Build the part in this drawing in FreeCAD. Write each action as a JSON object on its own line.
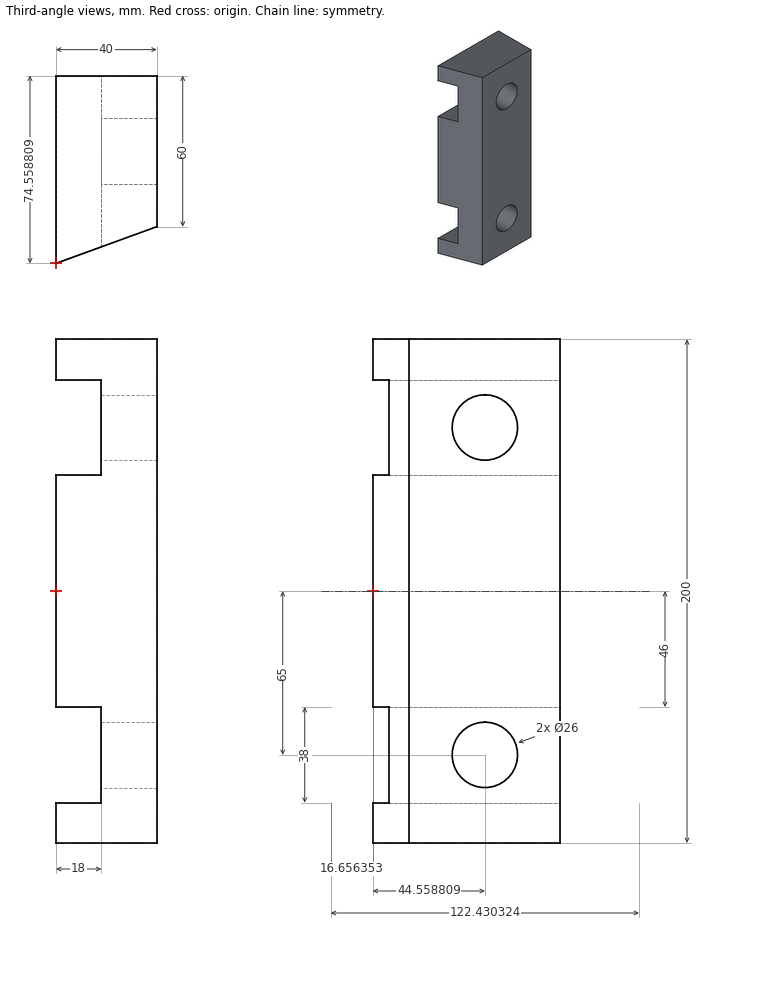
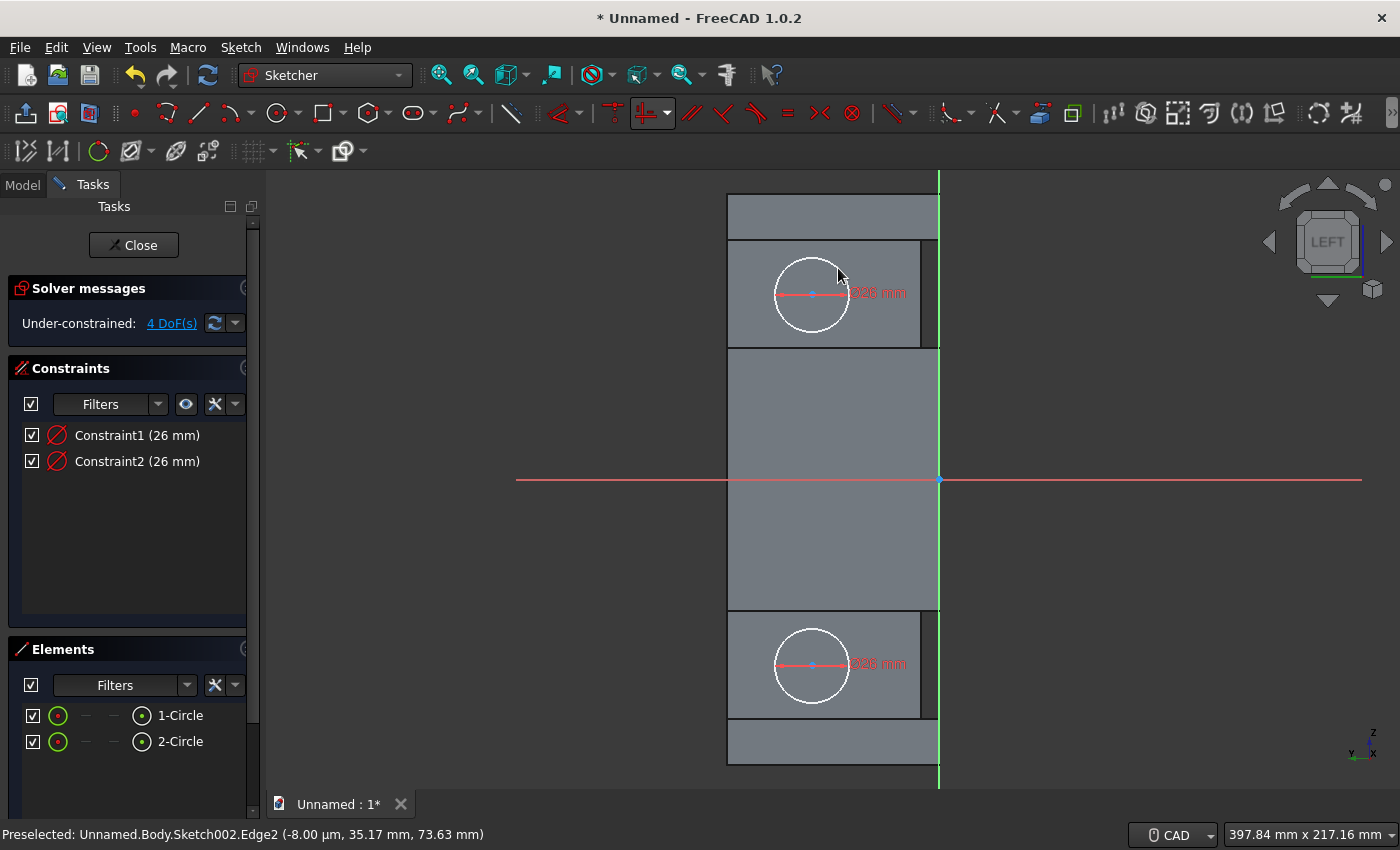
{"action": "left_click", "coordinate": [812, 666]}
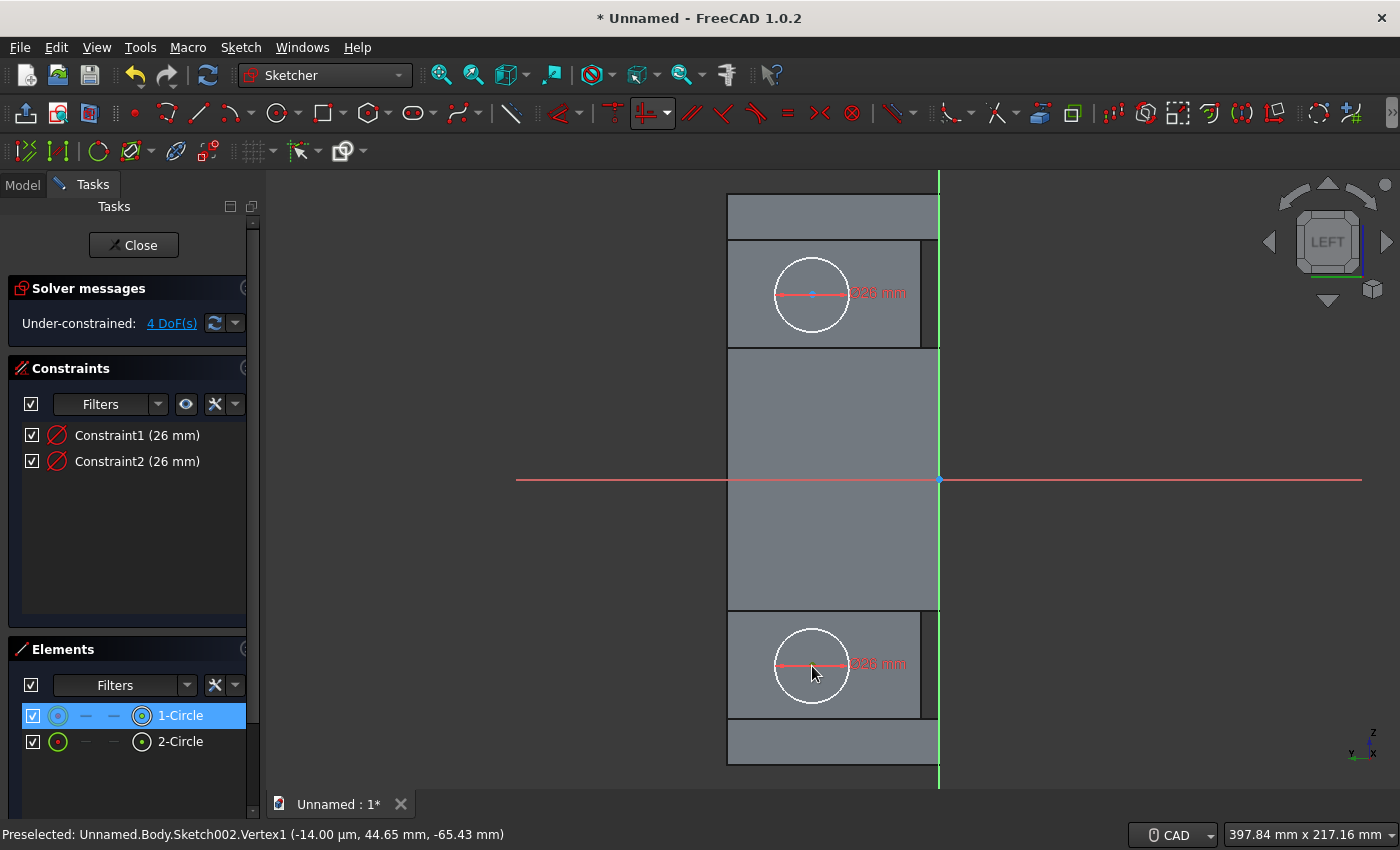
{"action": "left_click", "coordinate": [812, 295]}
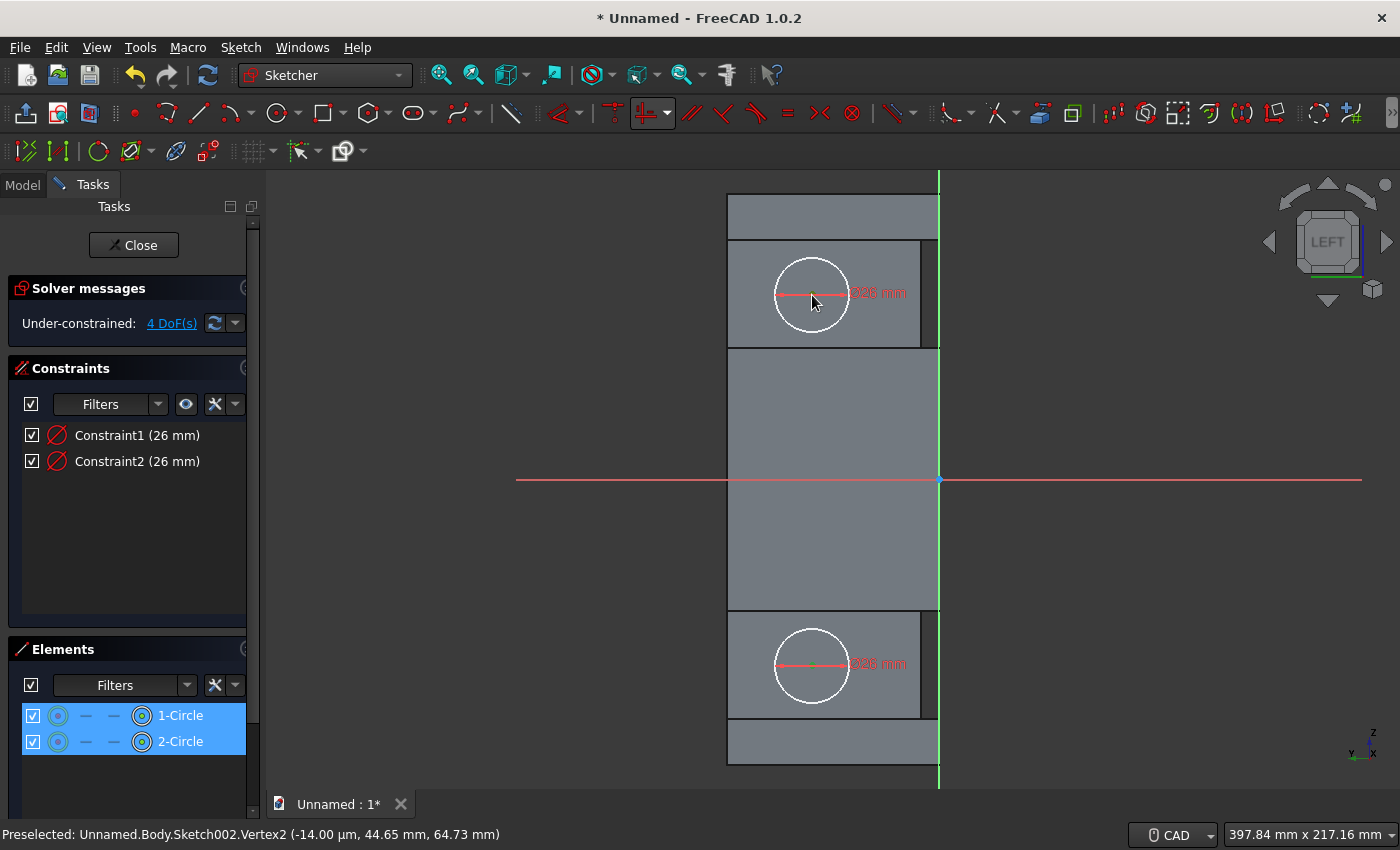
{"action": "left_click", "coordinate": [563, 480]}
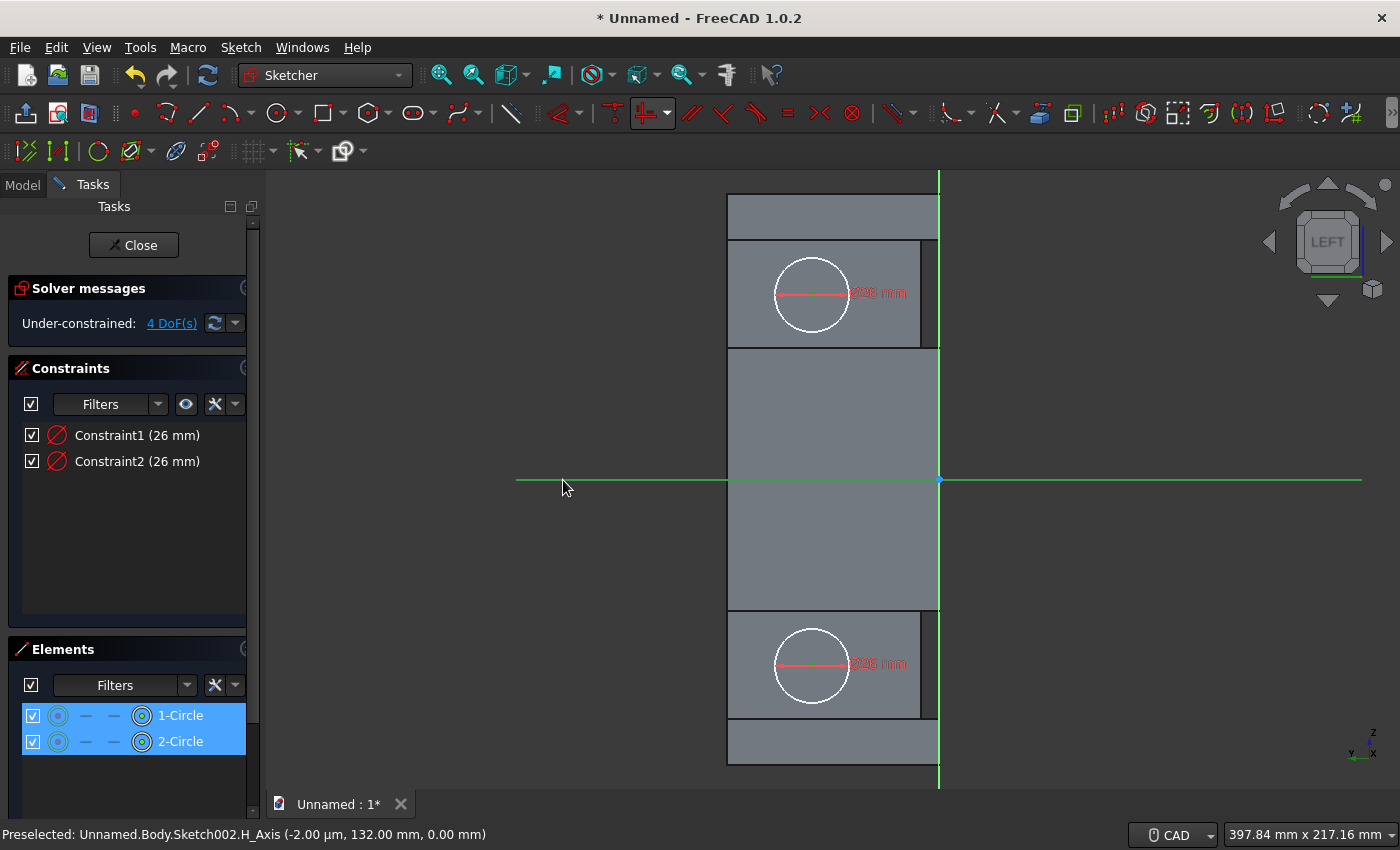
{"action": "left_click", "coordinate": [820, 114]}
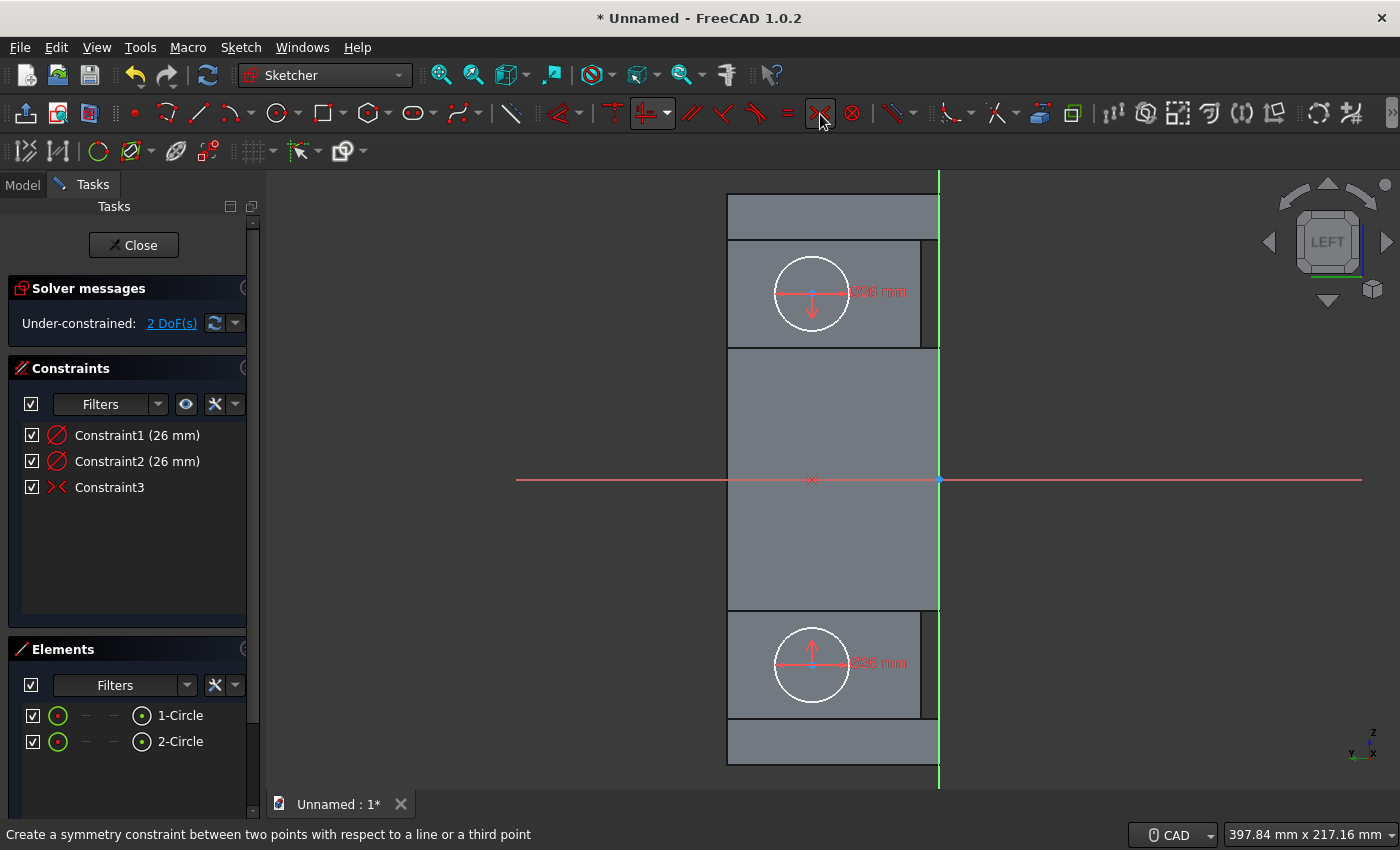
{"action": "left_click", "coordinate": [558, 114]}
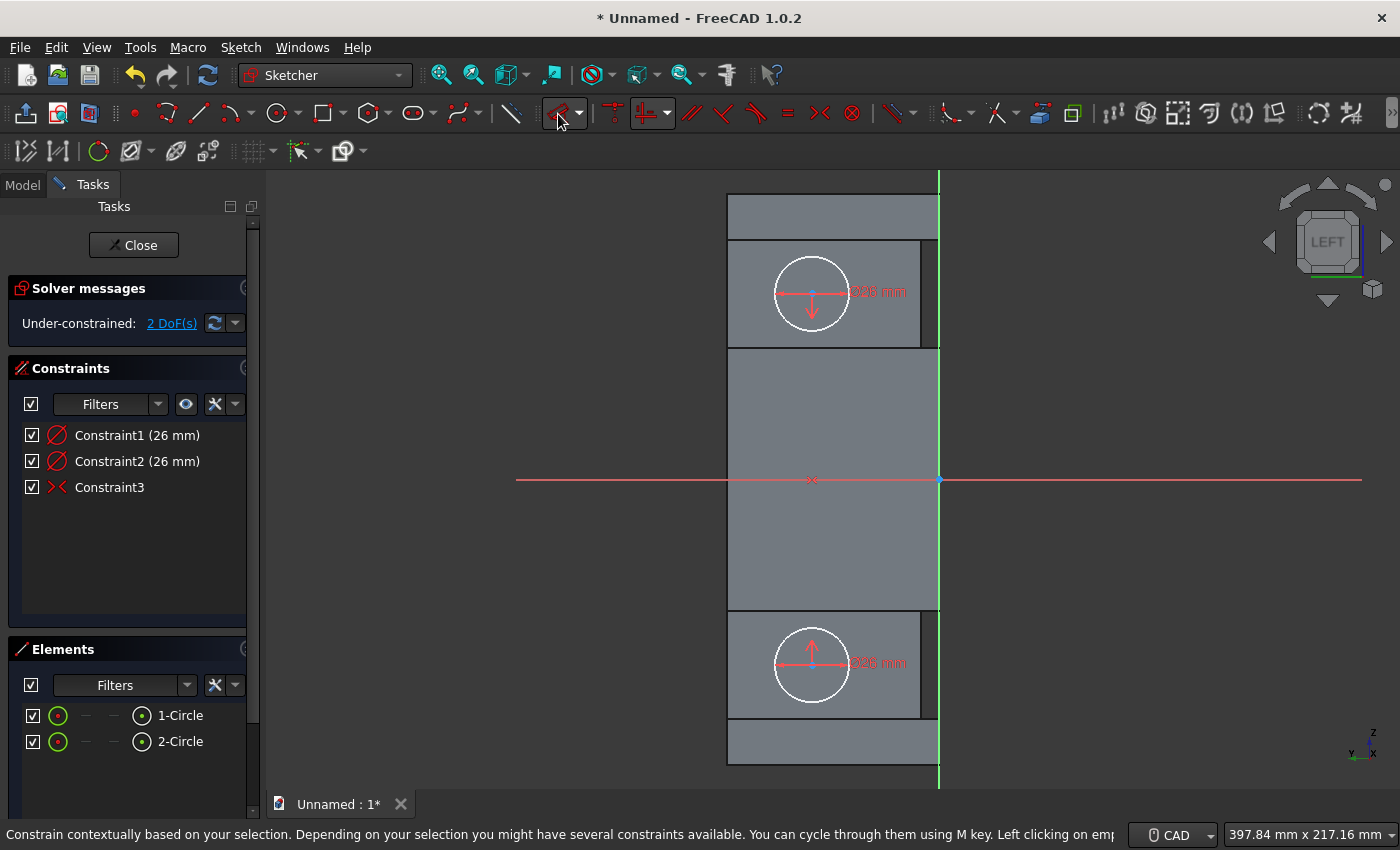
{"action": "left_click", "coordinate": [812, 665]}
{"action": "left_click", "coordinate": [973, 572]}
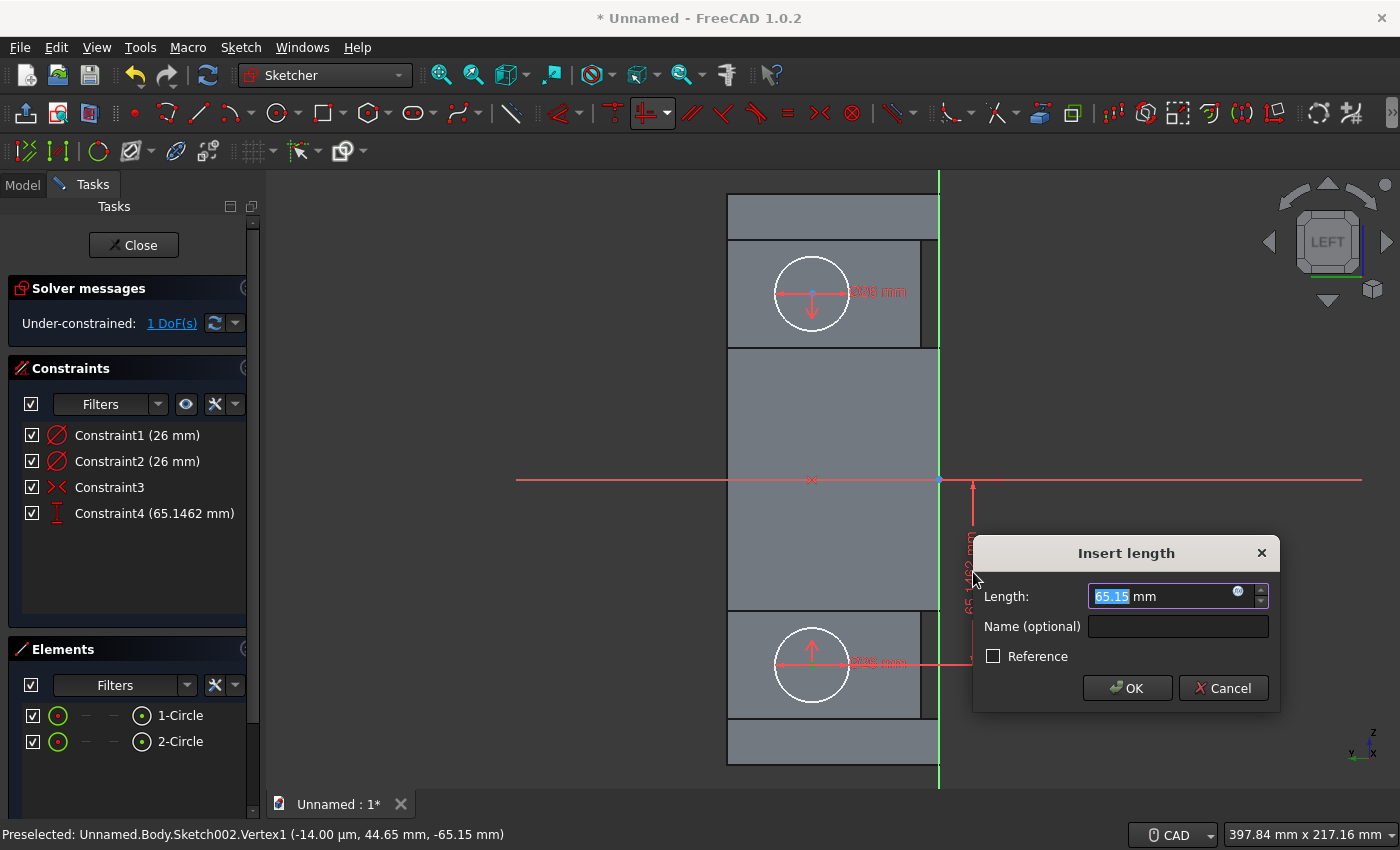
{"action": "type", "text": "65"}
{"action": "key", "text": "Return"}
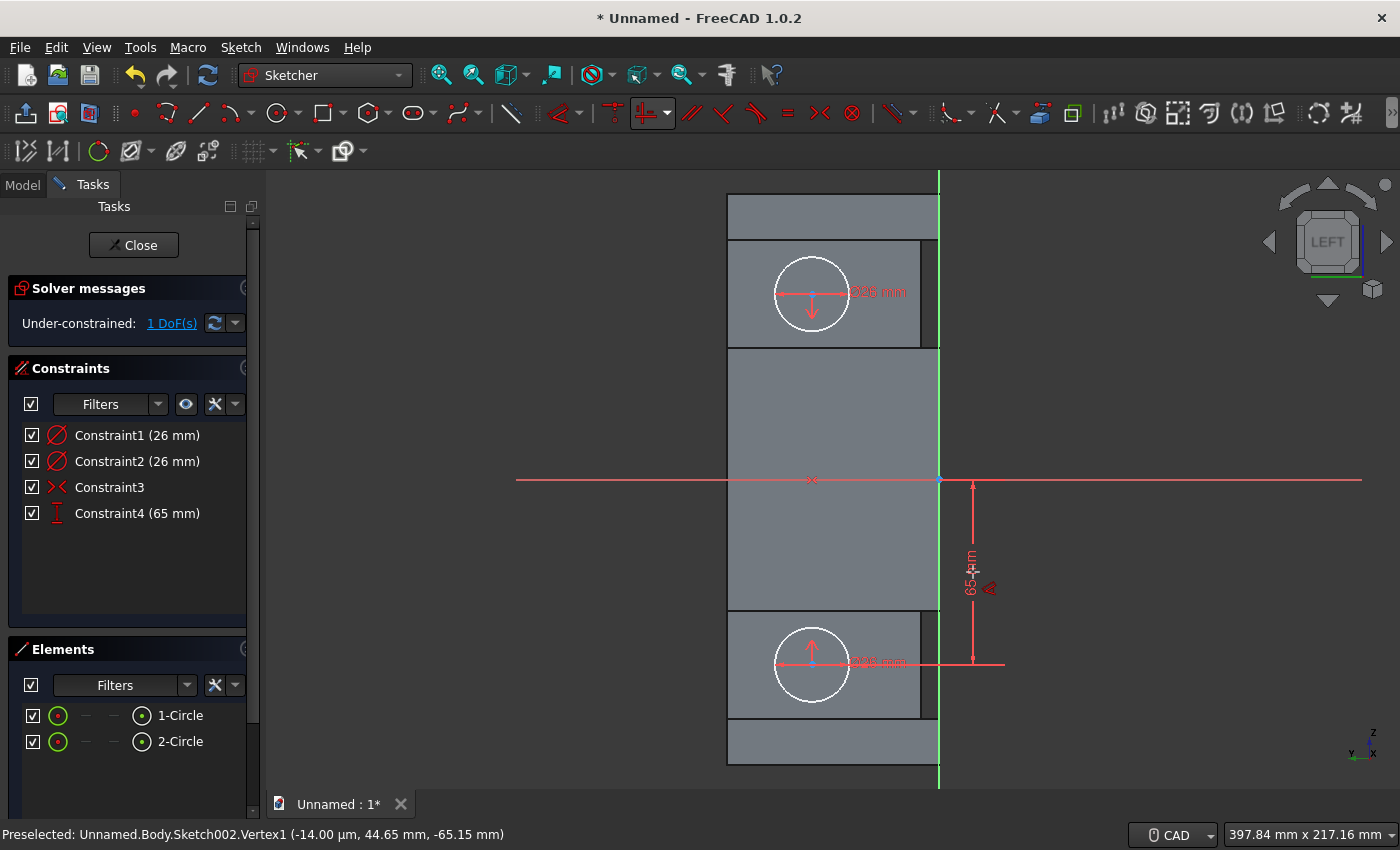
{"action": "left_click", "coordinate": [812, 665]}
{"action": "left_click", "coordinate": [876, 699]}